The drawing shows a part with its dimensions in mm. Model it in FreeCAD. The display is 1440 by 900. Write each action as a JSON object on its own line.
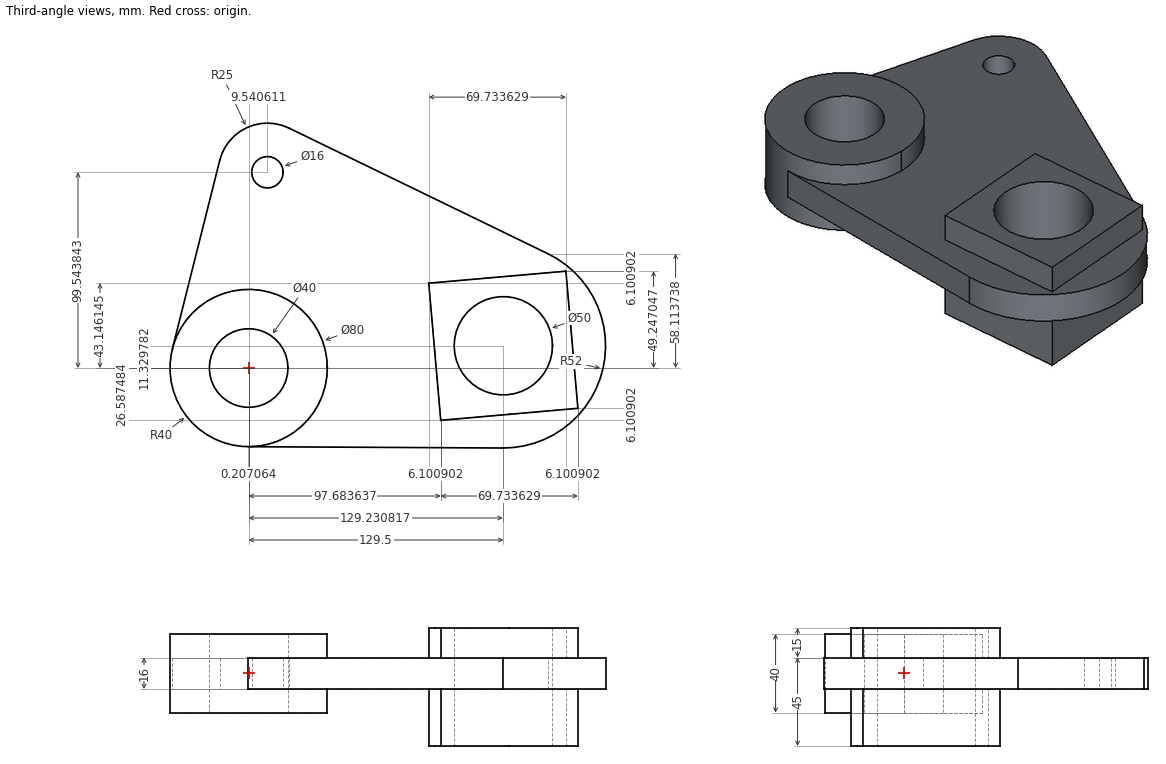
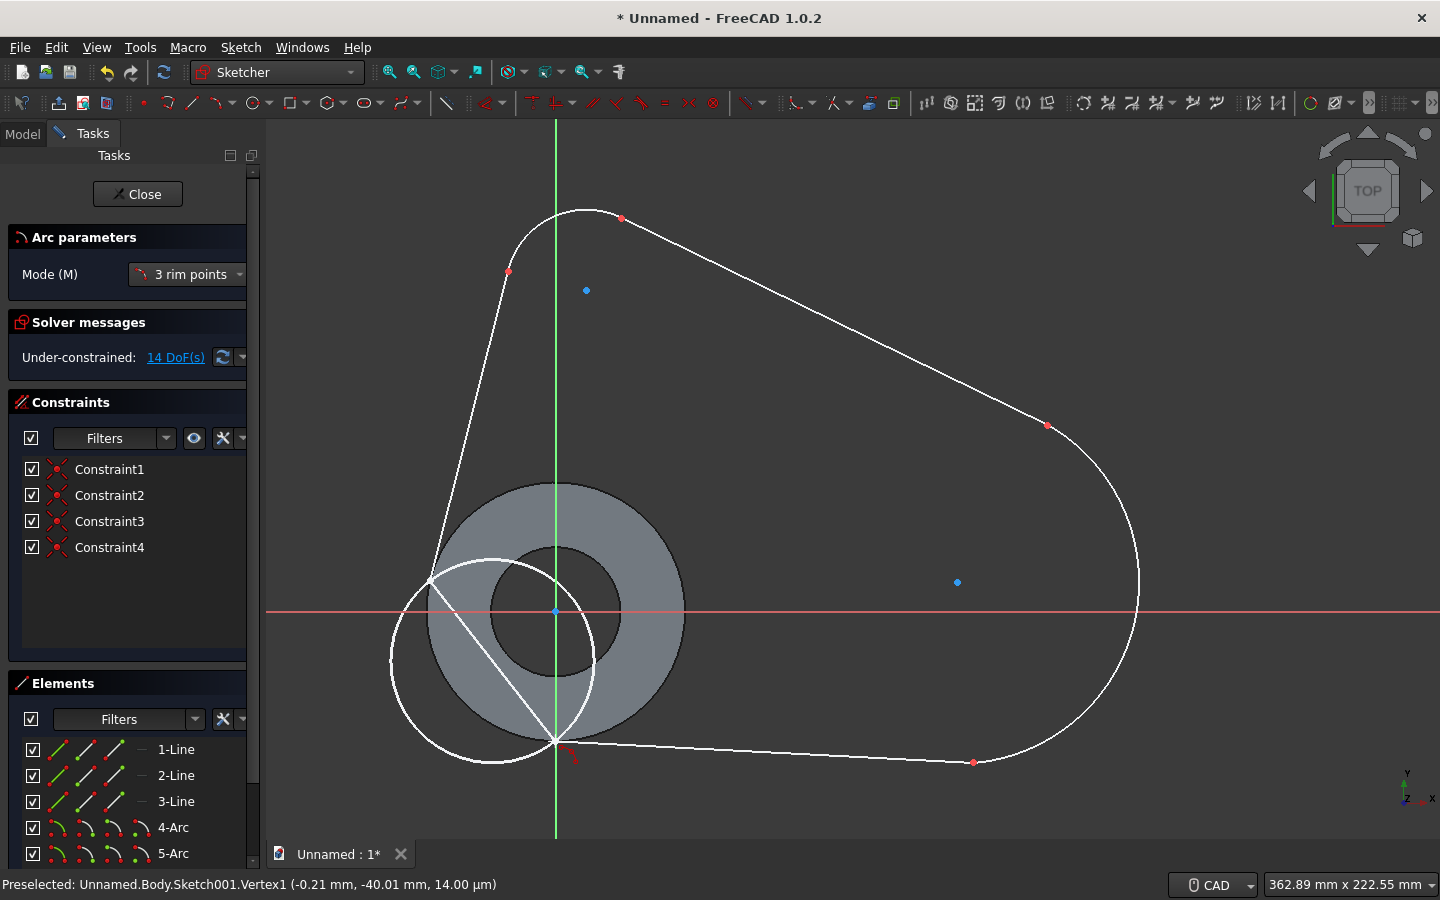
{"action": "left_click", "coordinate": [454, 691]}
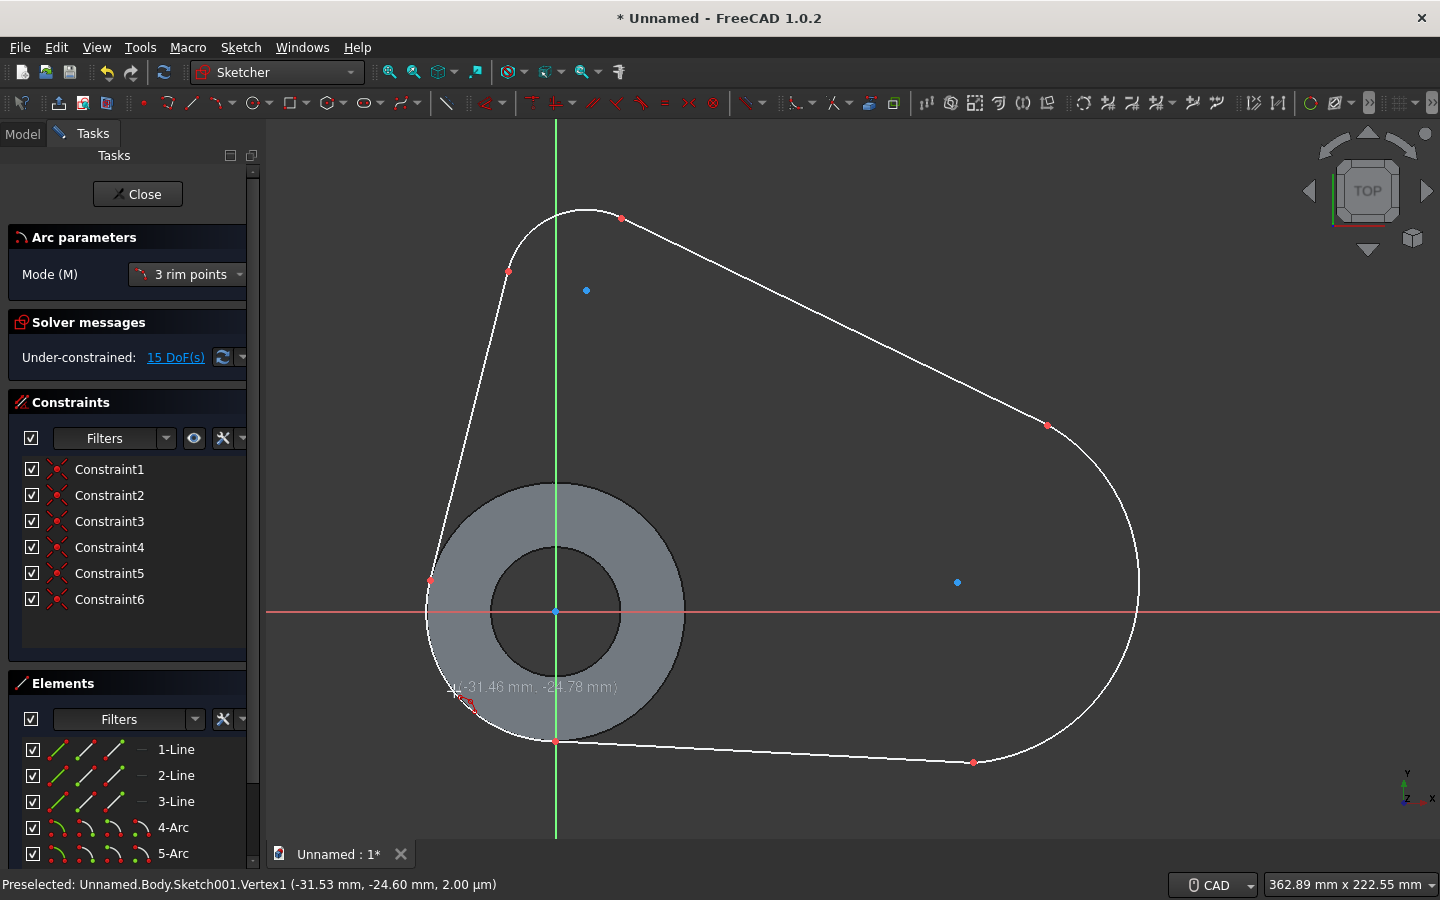
{"action": "left_click", "coordinate": [168, 104]}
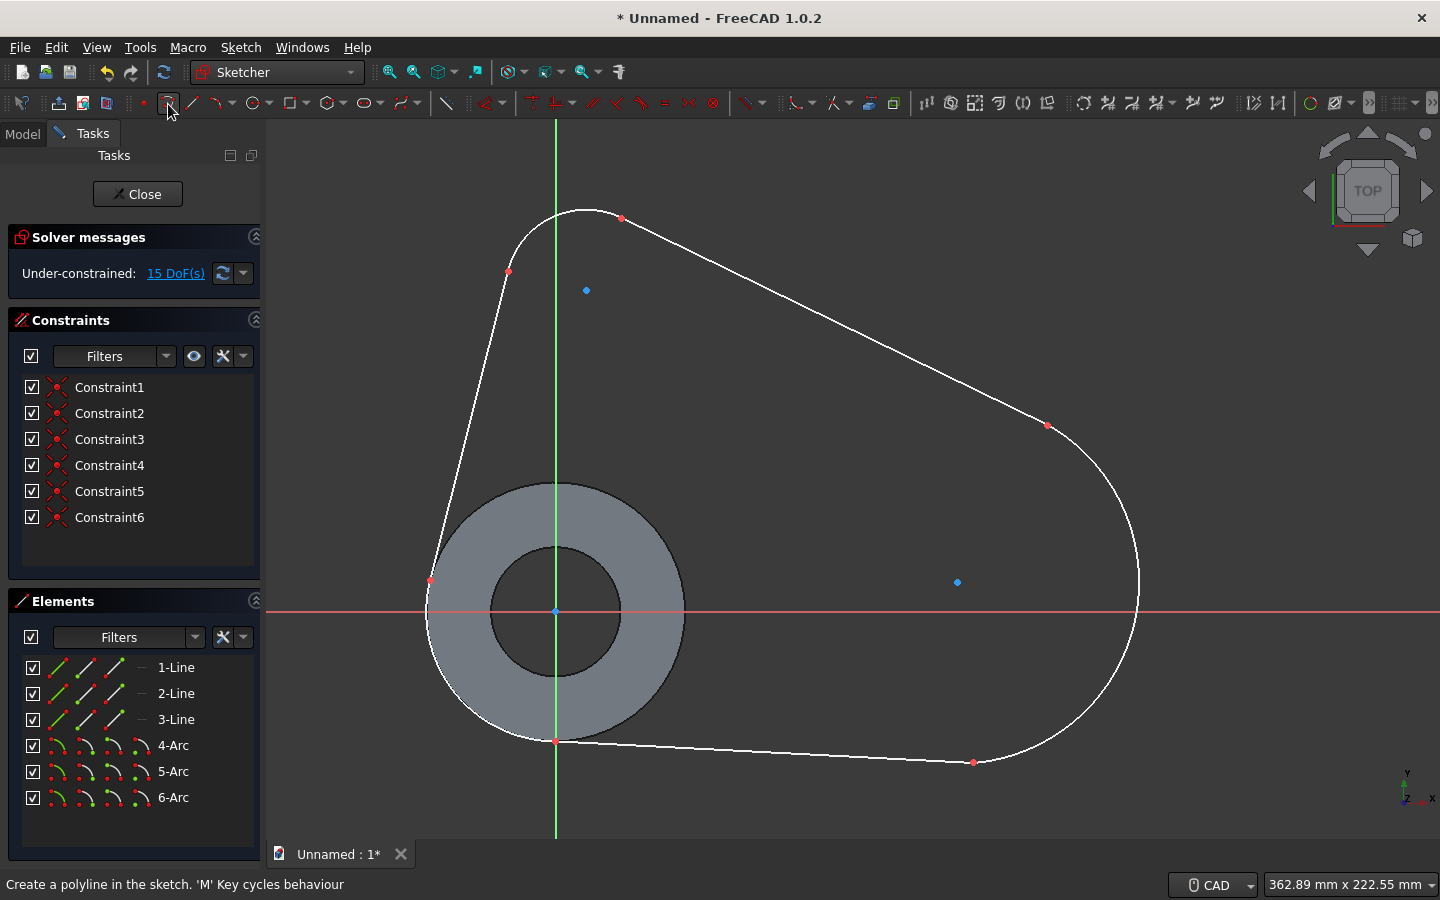
{"action": "left_click", "coordinate": [872, 698]}
{"action": "left_click", "coordinate": [852, 472]}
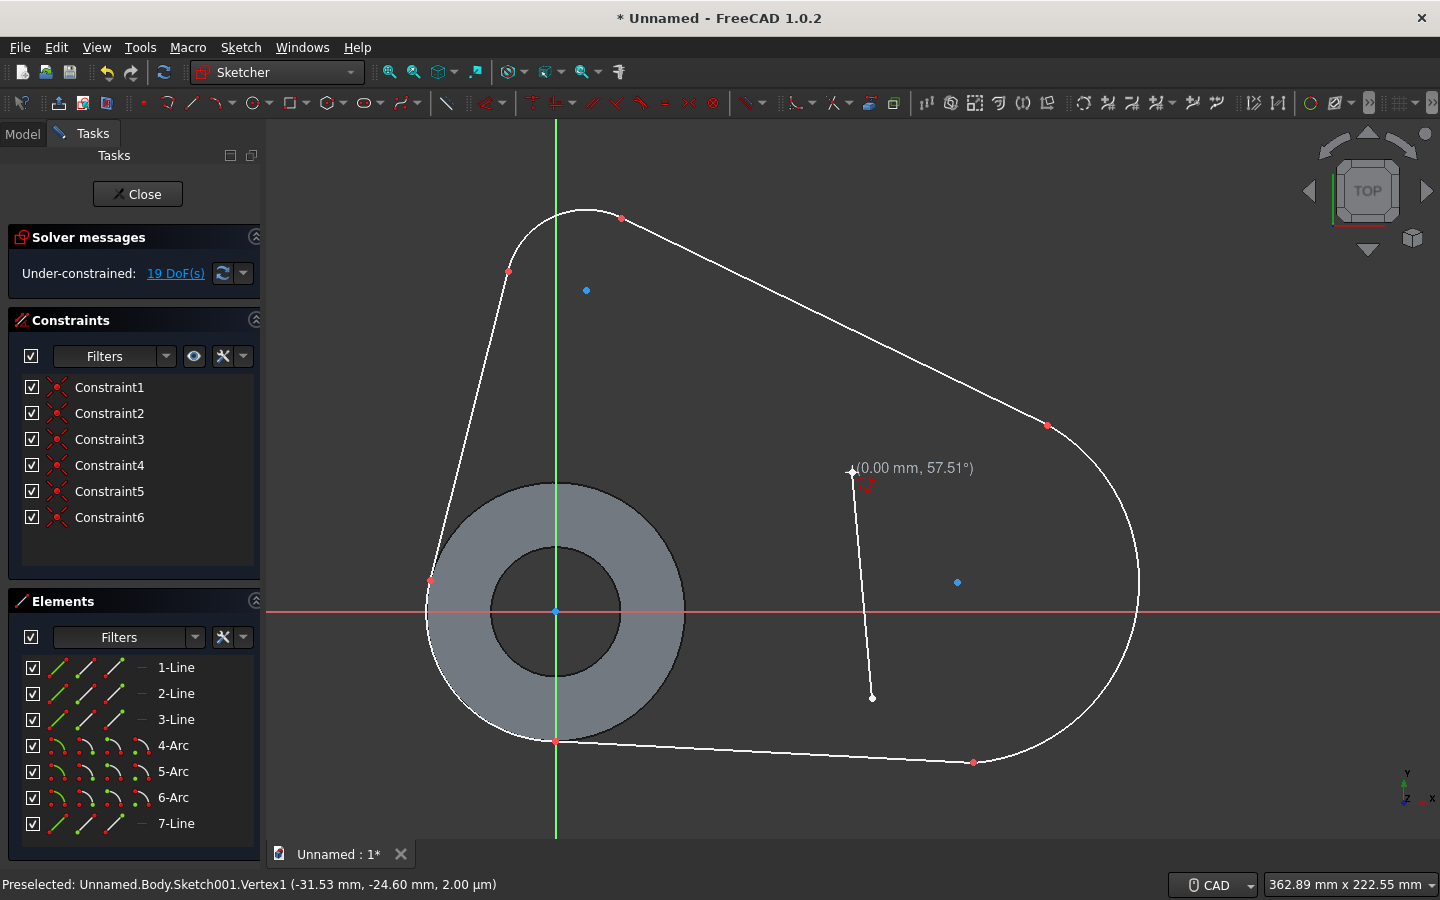
{"action": "scroll", "coordinate": [1078, 453], "scroll_direction": "up", "scroll_amount": 4}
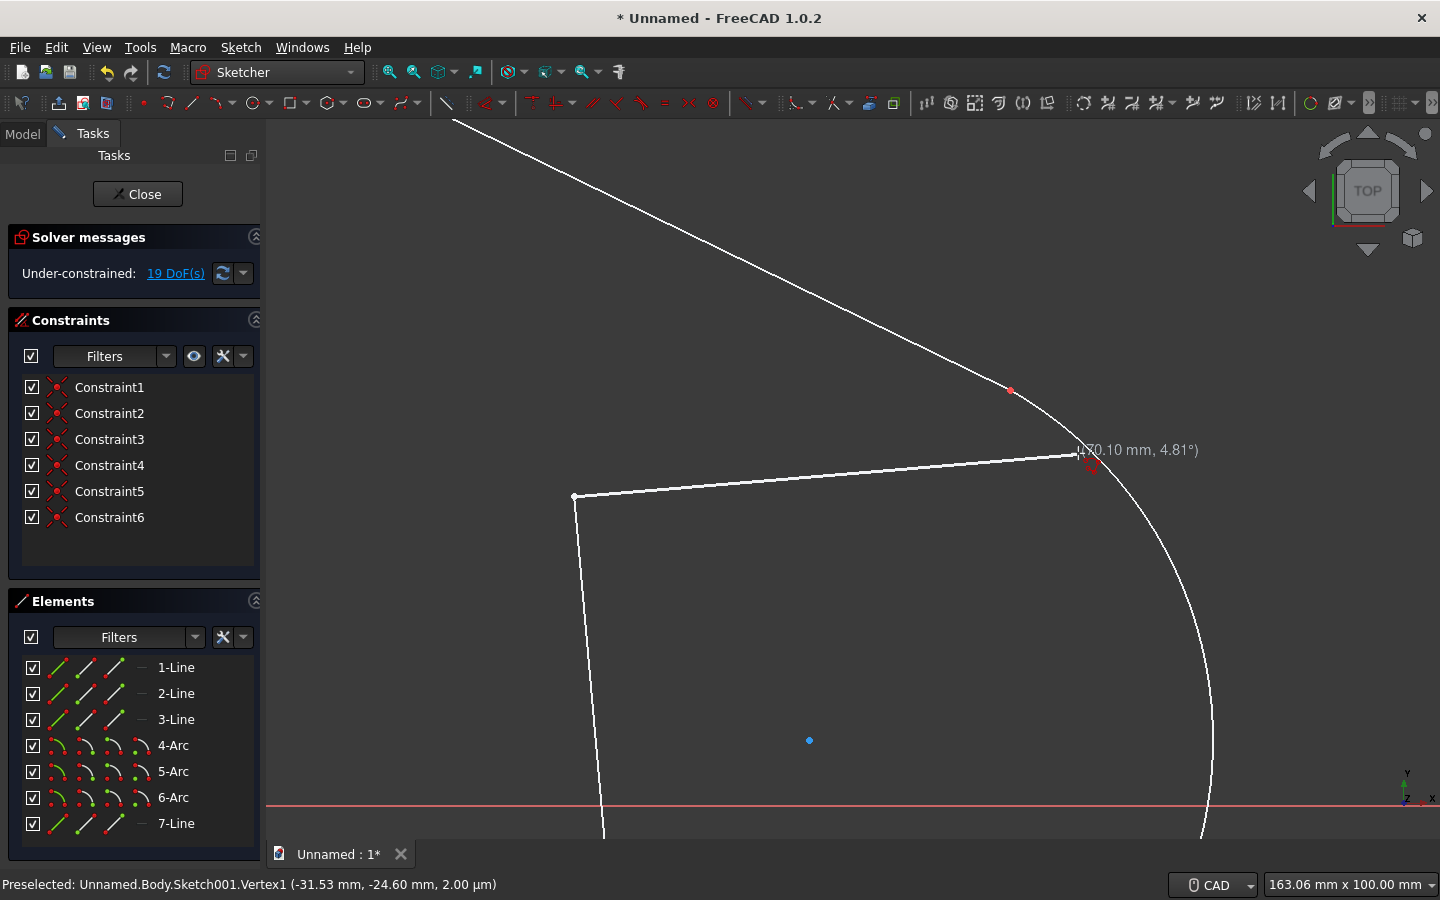
{"action": "left_click", "coordinate": [1076, 451]}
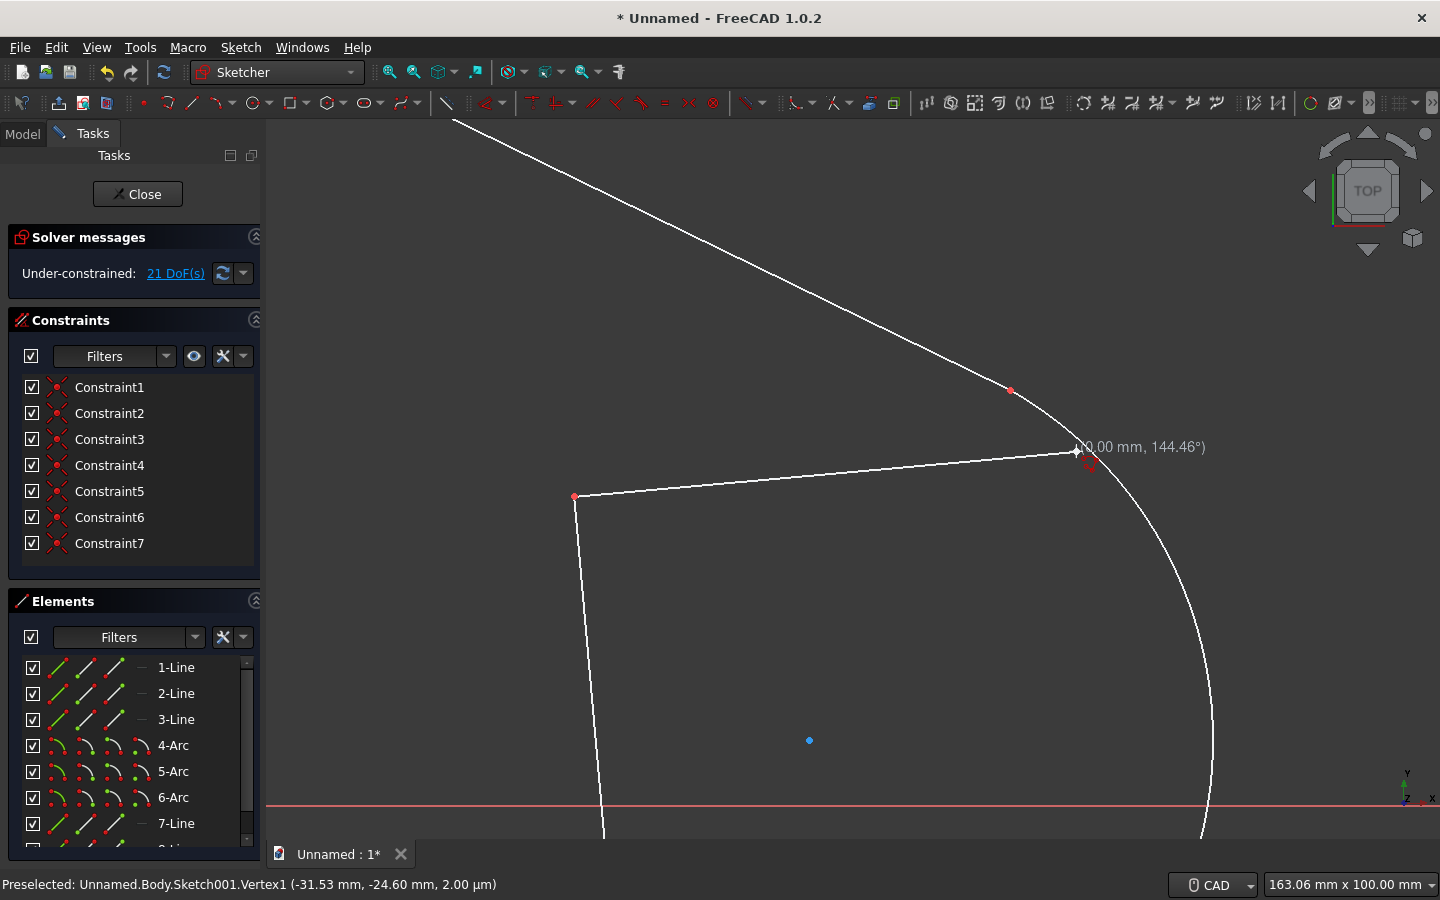
{"action": "scroll", "coordinate": [994, 460], "scroll_direction": "down", "scroll_amount": 5}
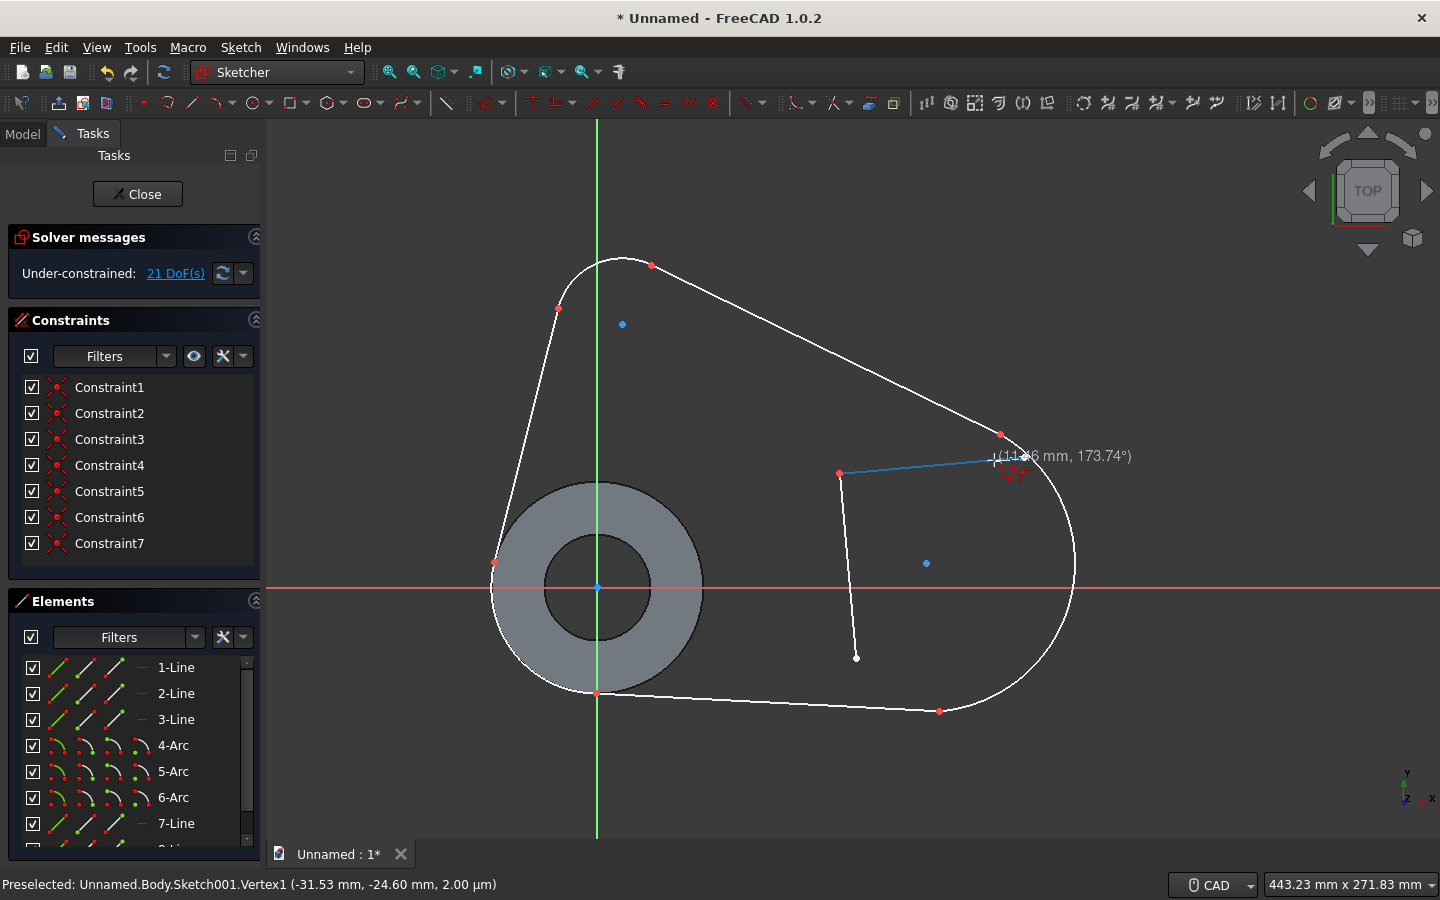
{"action": "scroll", "coordinate": [1041, 642], "scroll_direction": "up", "scroll_amount": 5}